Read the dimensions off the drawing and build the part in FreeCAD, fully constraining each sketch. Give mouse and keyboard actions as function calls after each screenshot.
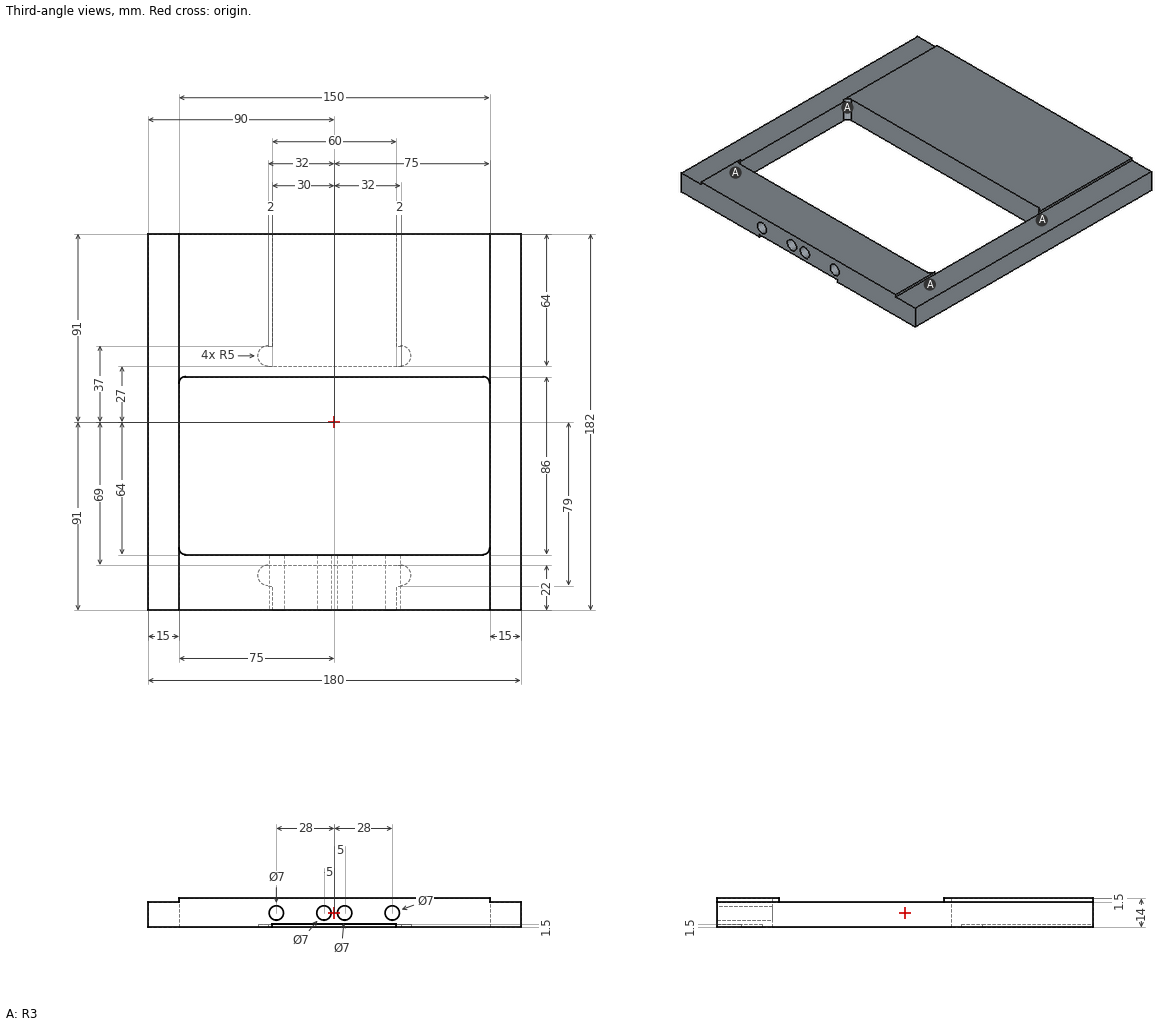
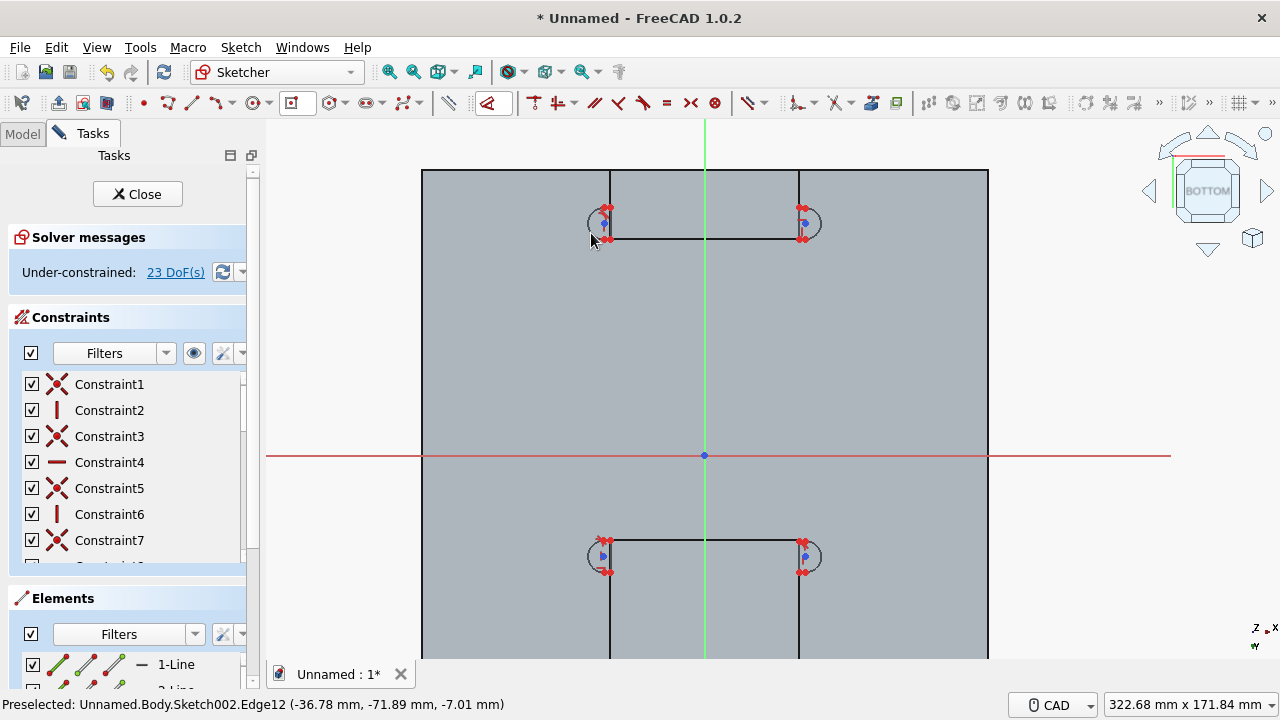
scroll(607, 208, up, 8)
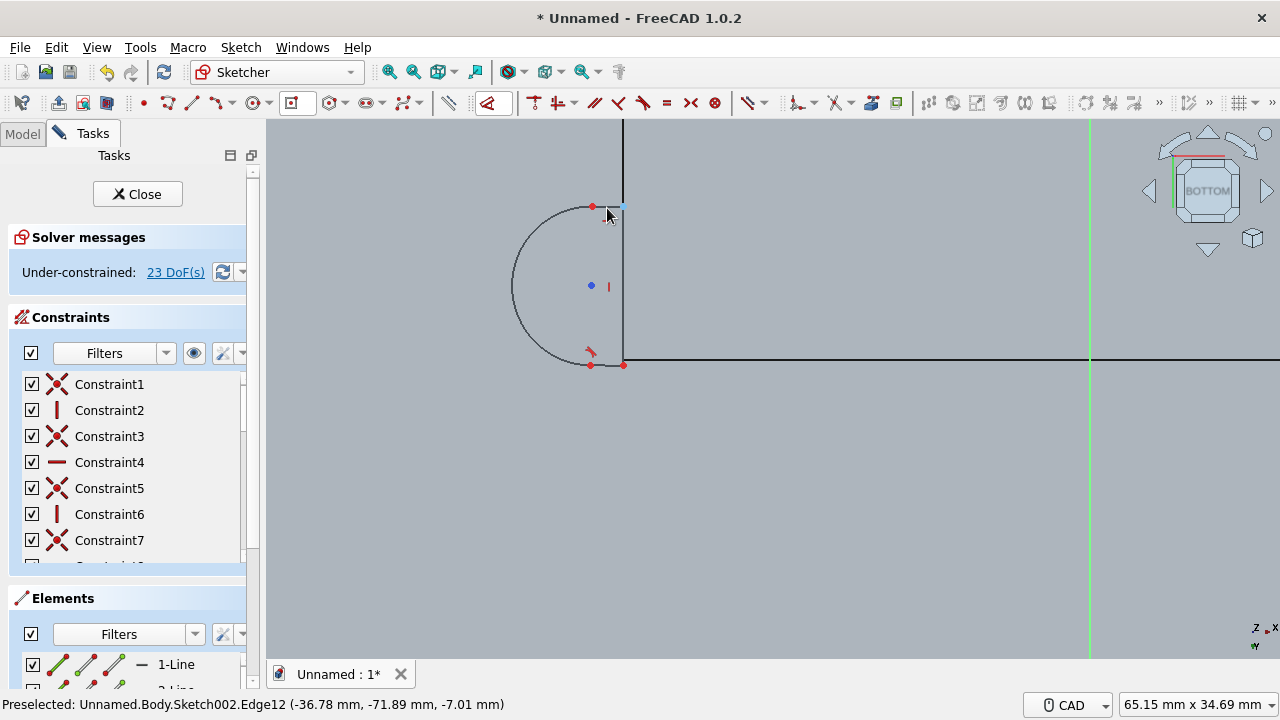
click(608, 207)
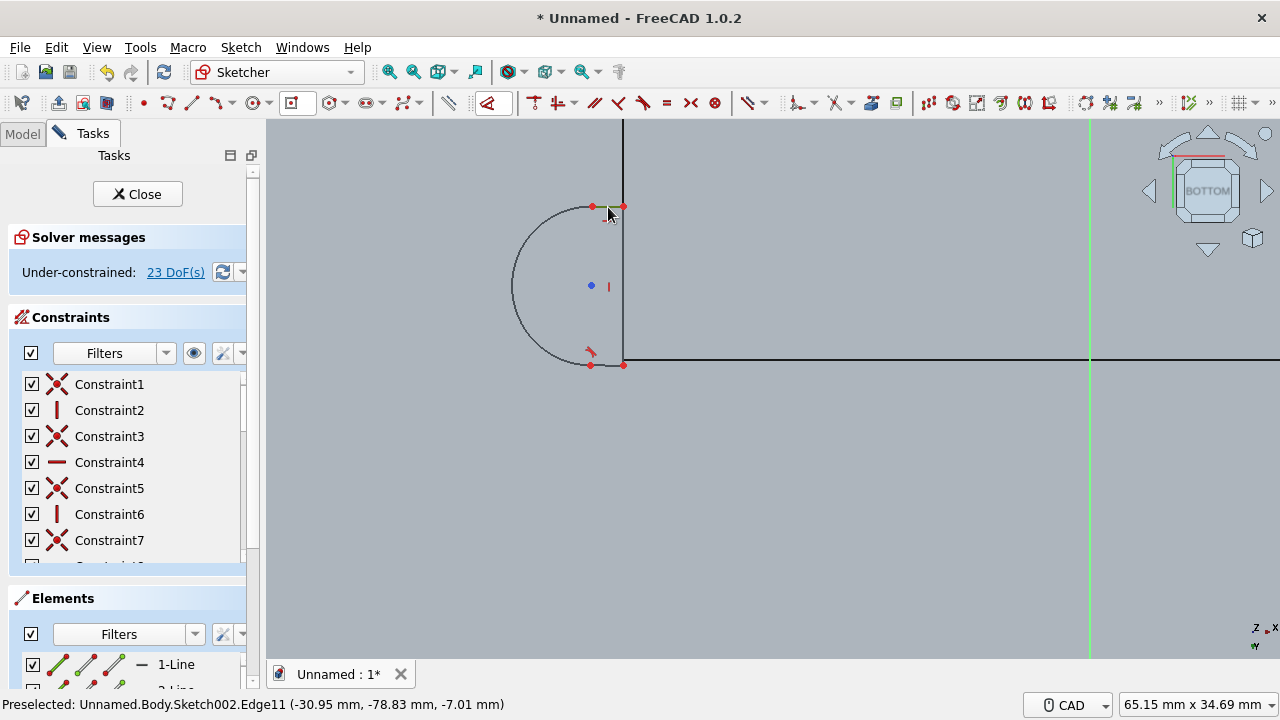
scroll(607, 207, down, 8)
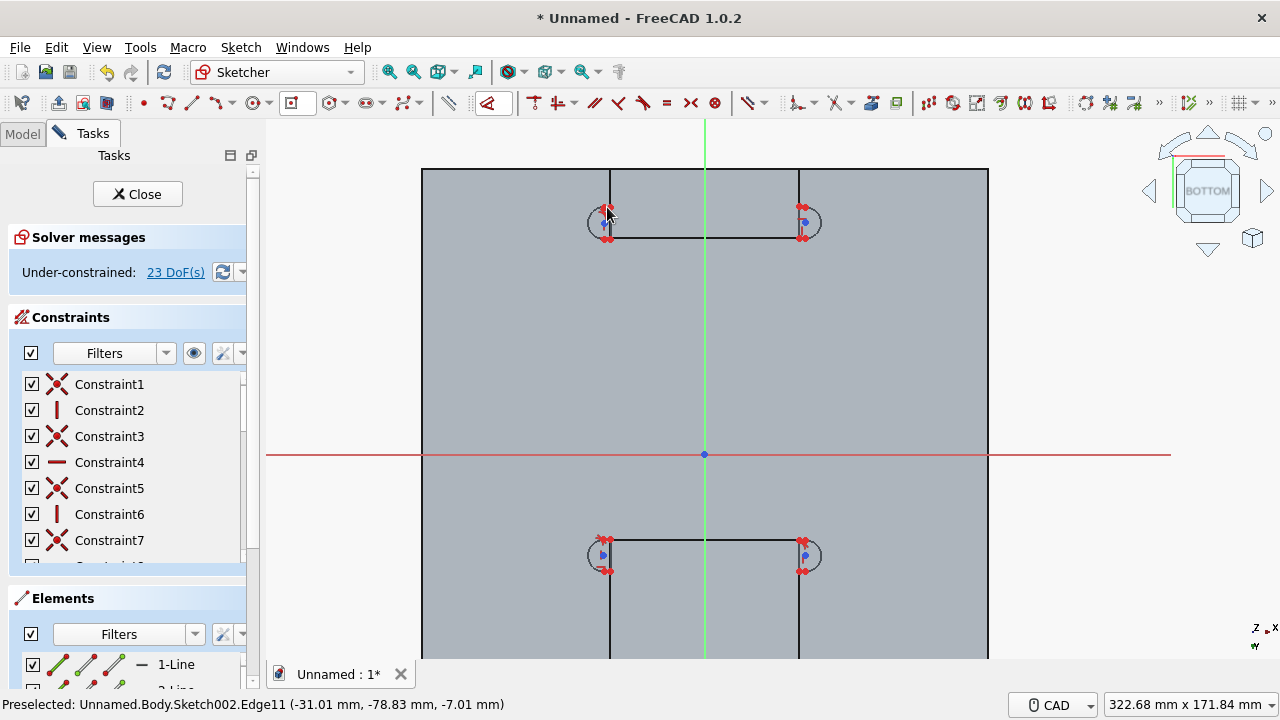
click(591, 214)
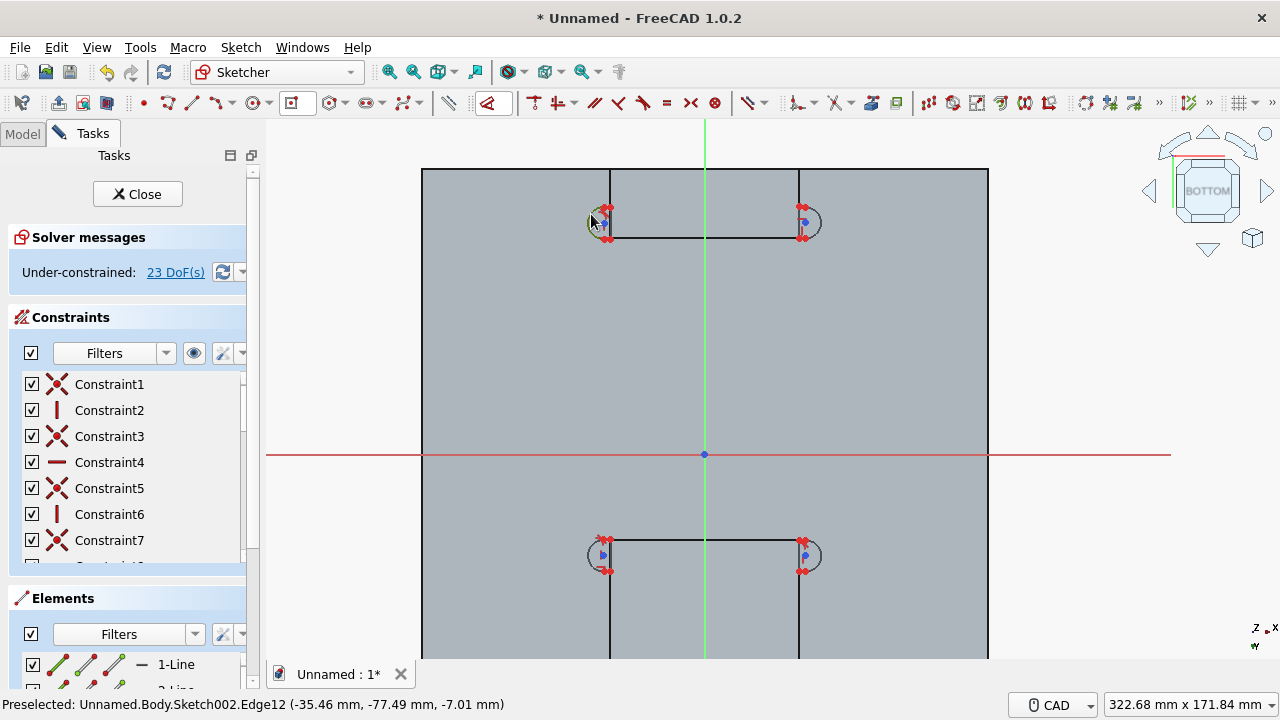
key(t)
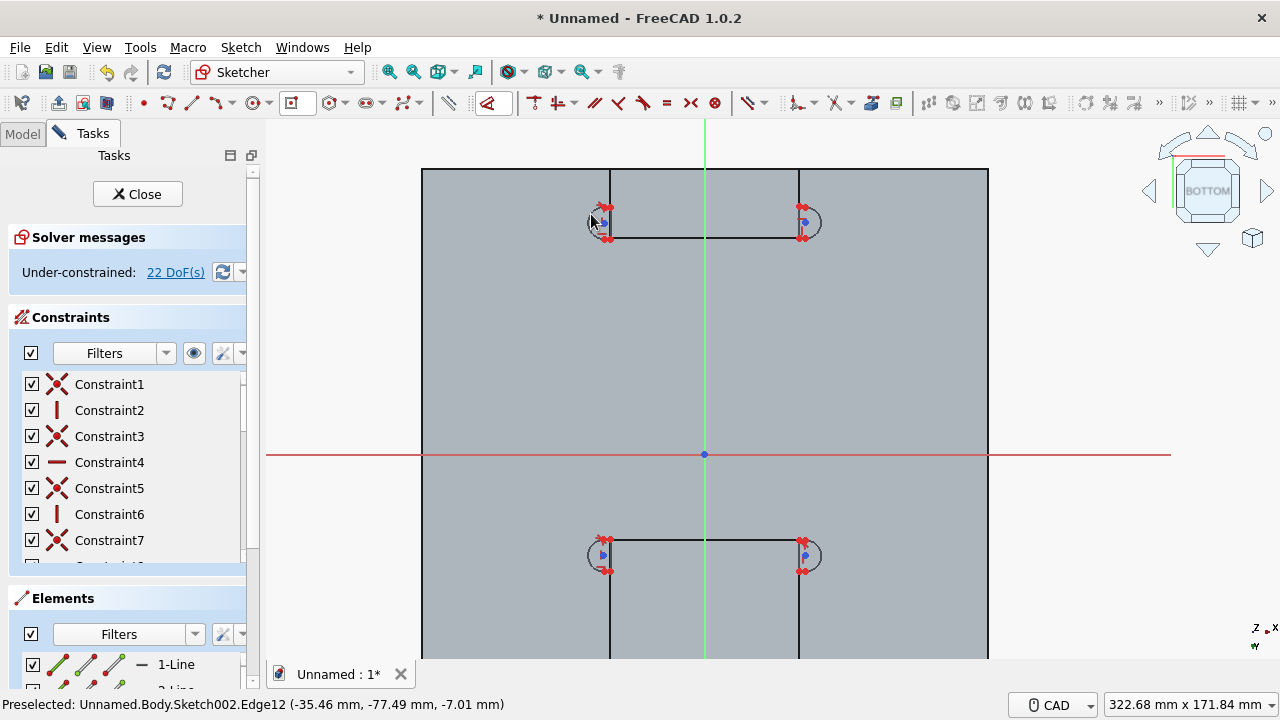
scroll(802, 207, up, 8)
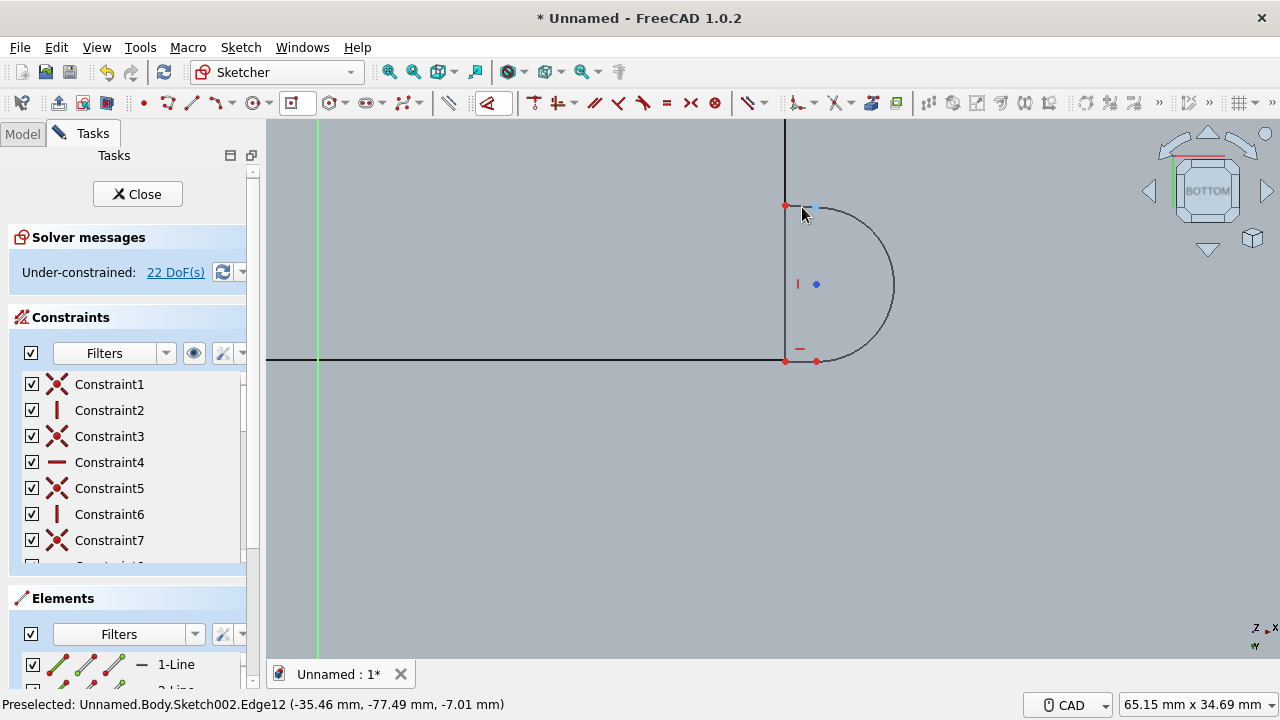
click(800, 206)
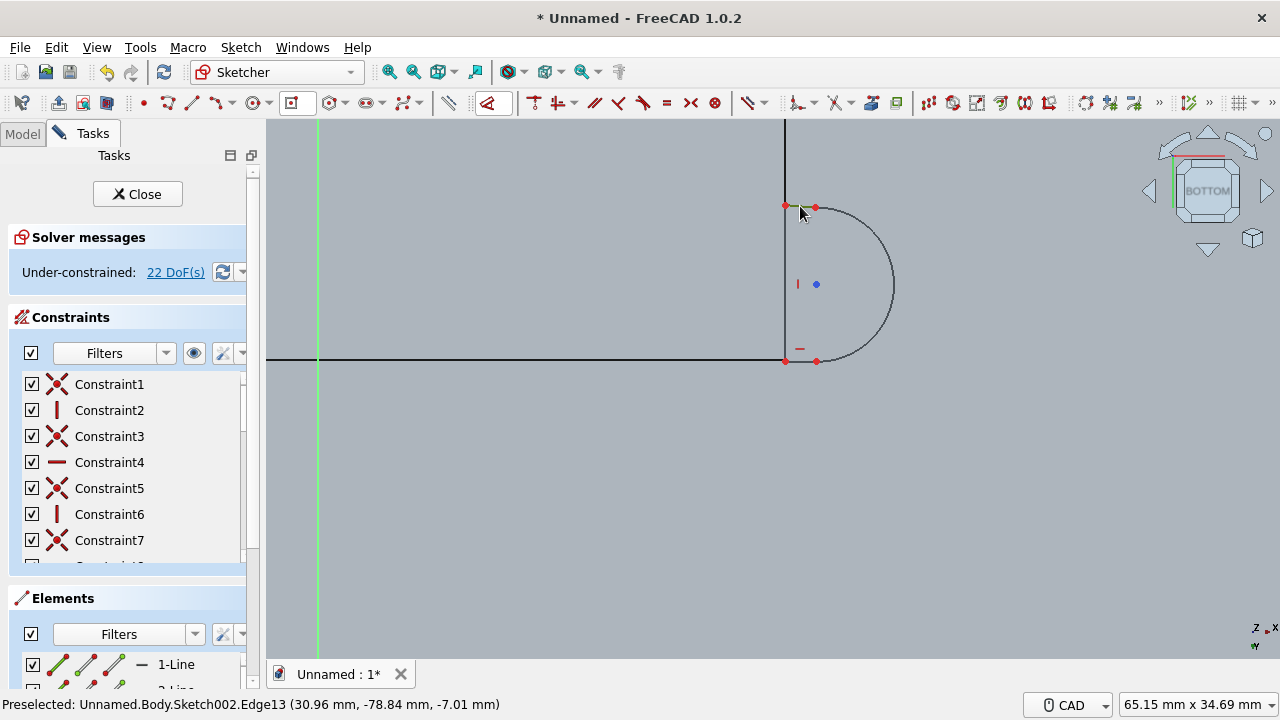
scroll(802, 207, down, 8)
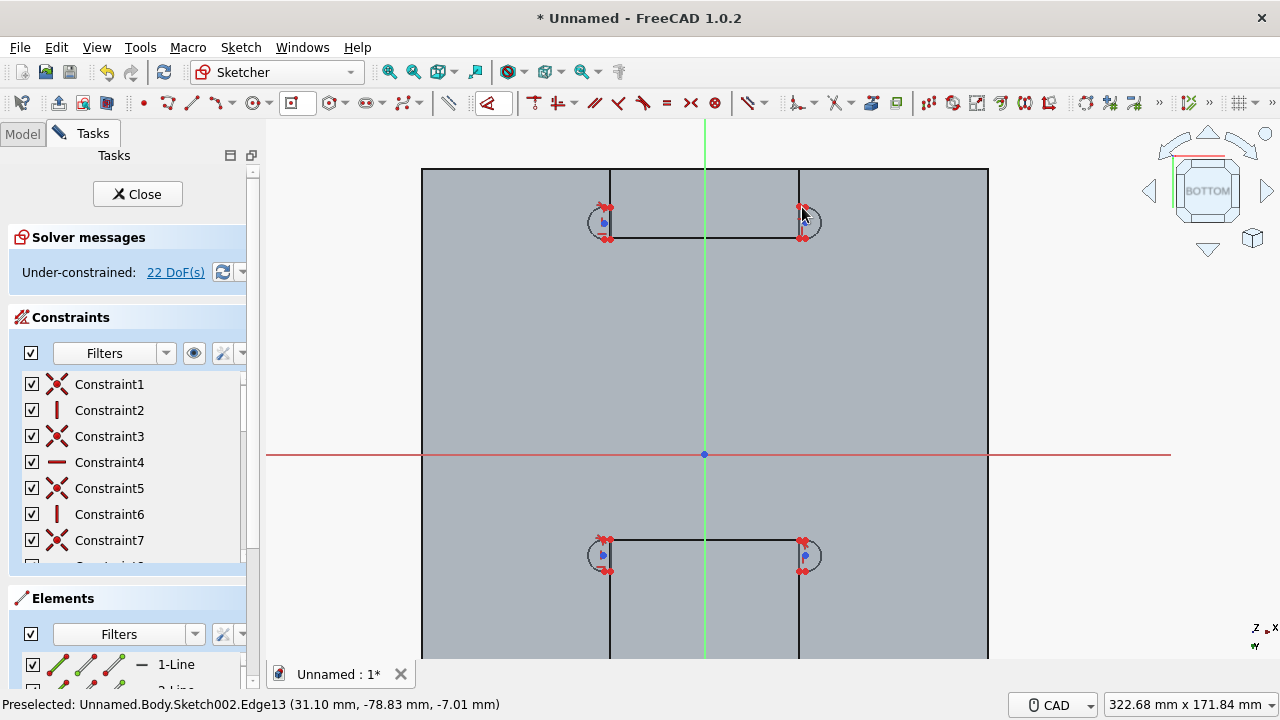
click(818, 232)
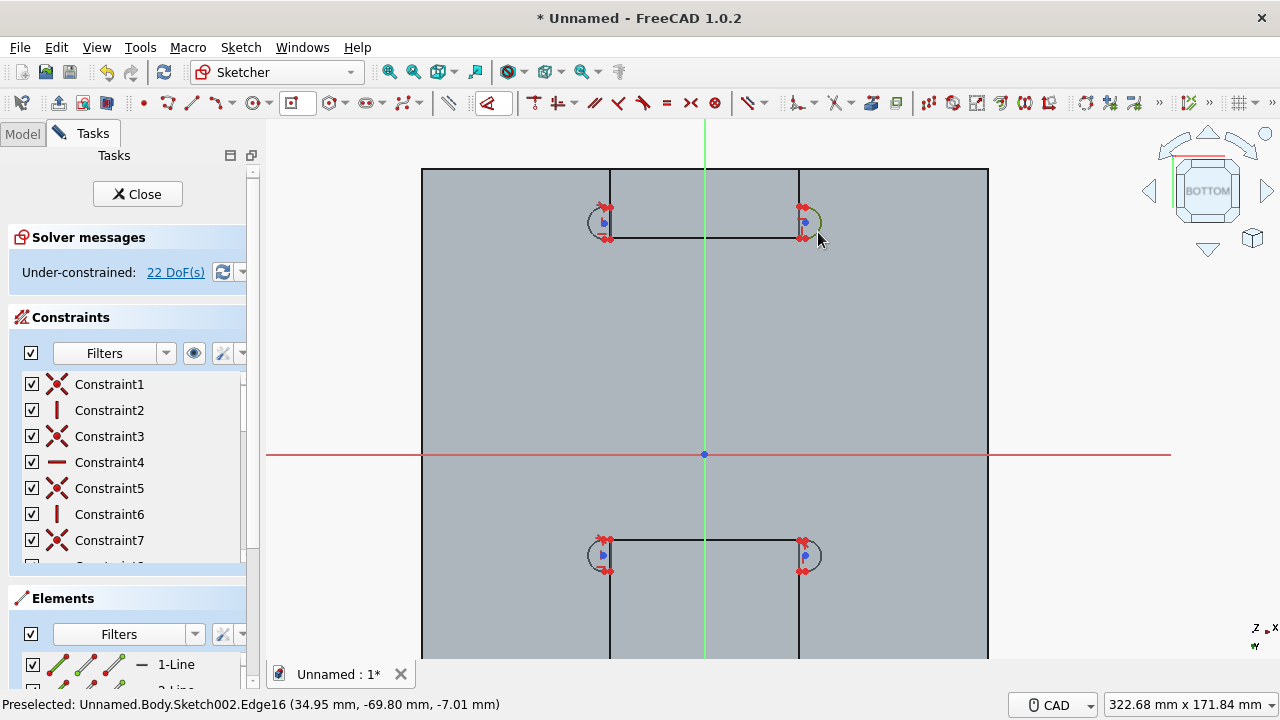
key(t)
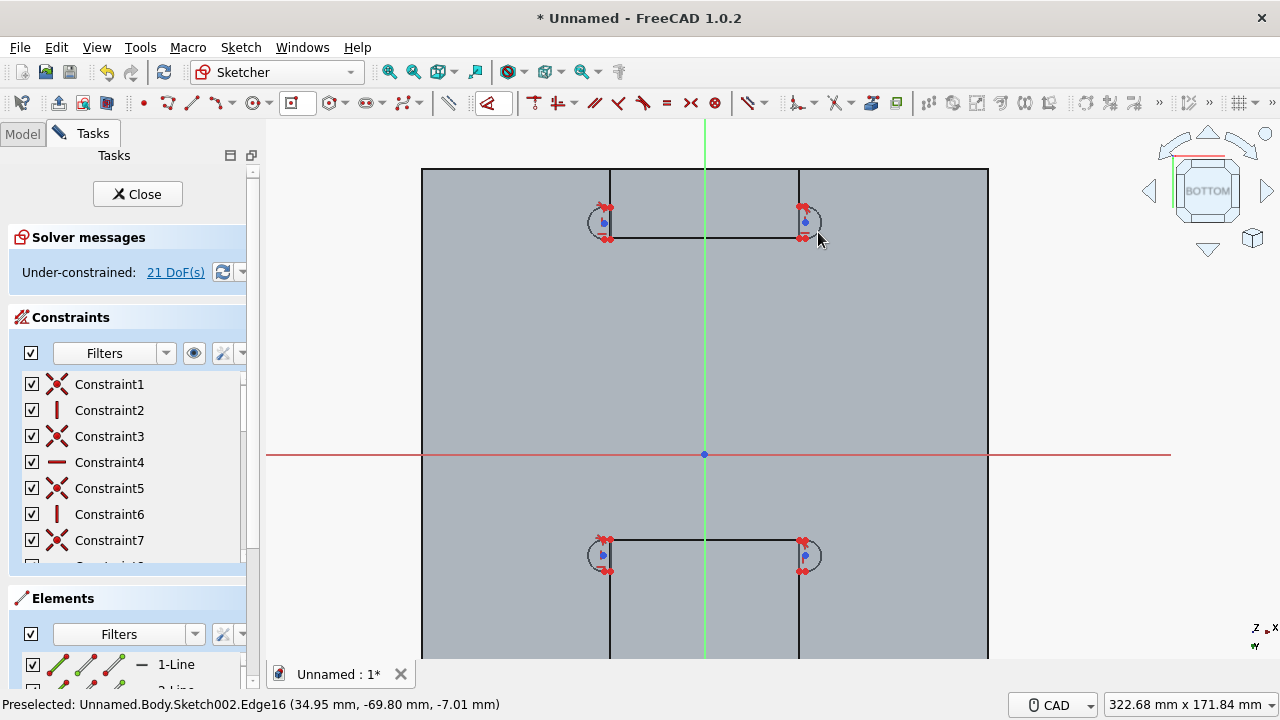
scroll(802, 238, up, 8)